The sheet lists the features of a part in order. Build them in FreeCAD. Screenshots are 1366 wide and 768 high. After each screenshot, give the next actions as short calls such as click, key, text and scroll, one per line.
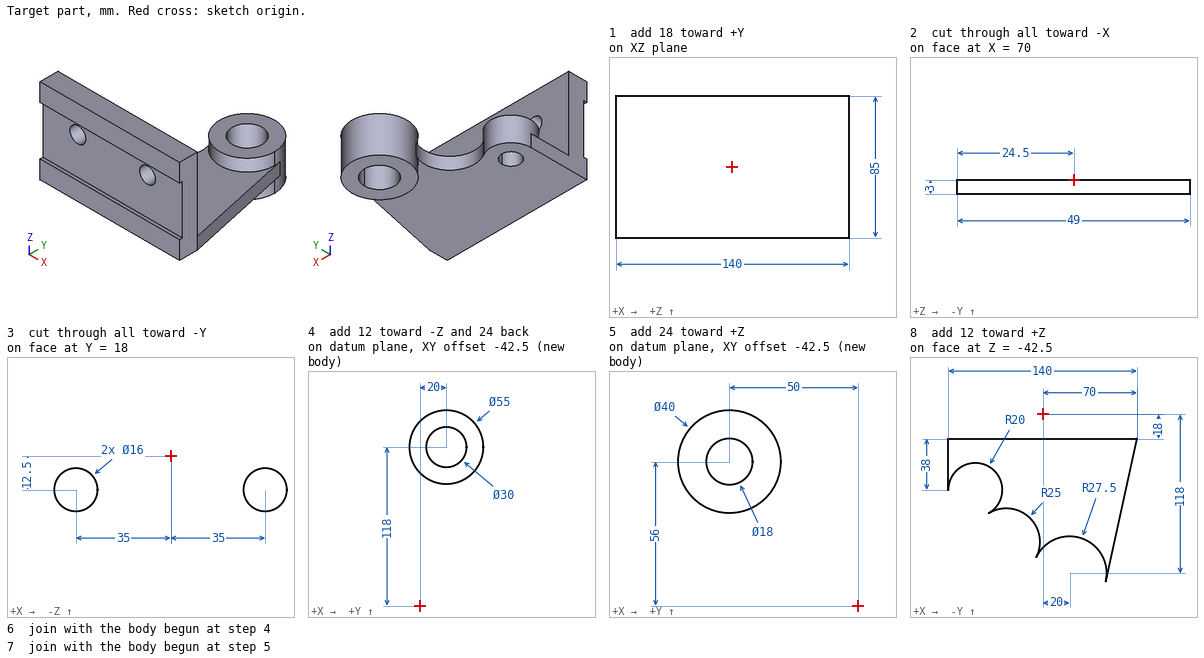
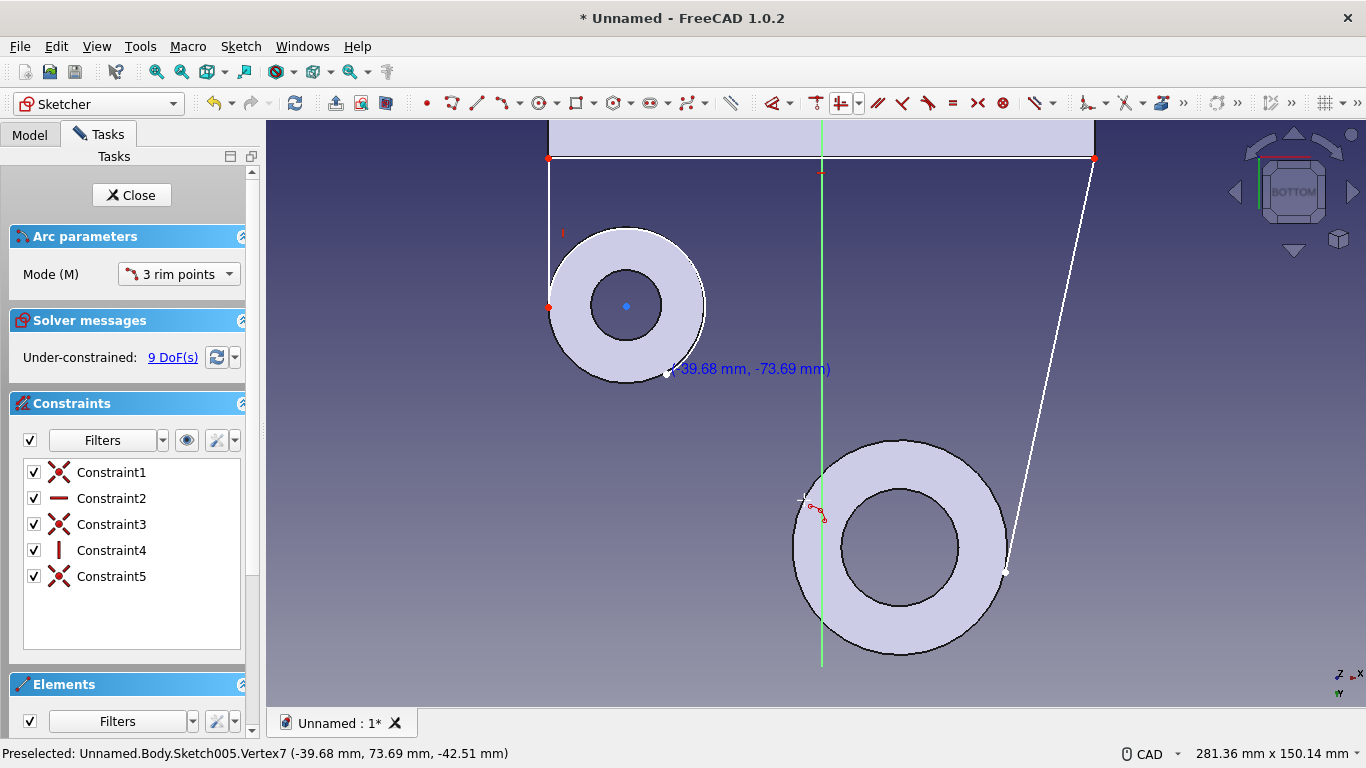
click(803, 500)
click(782, 385)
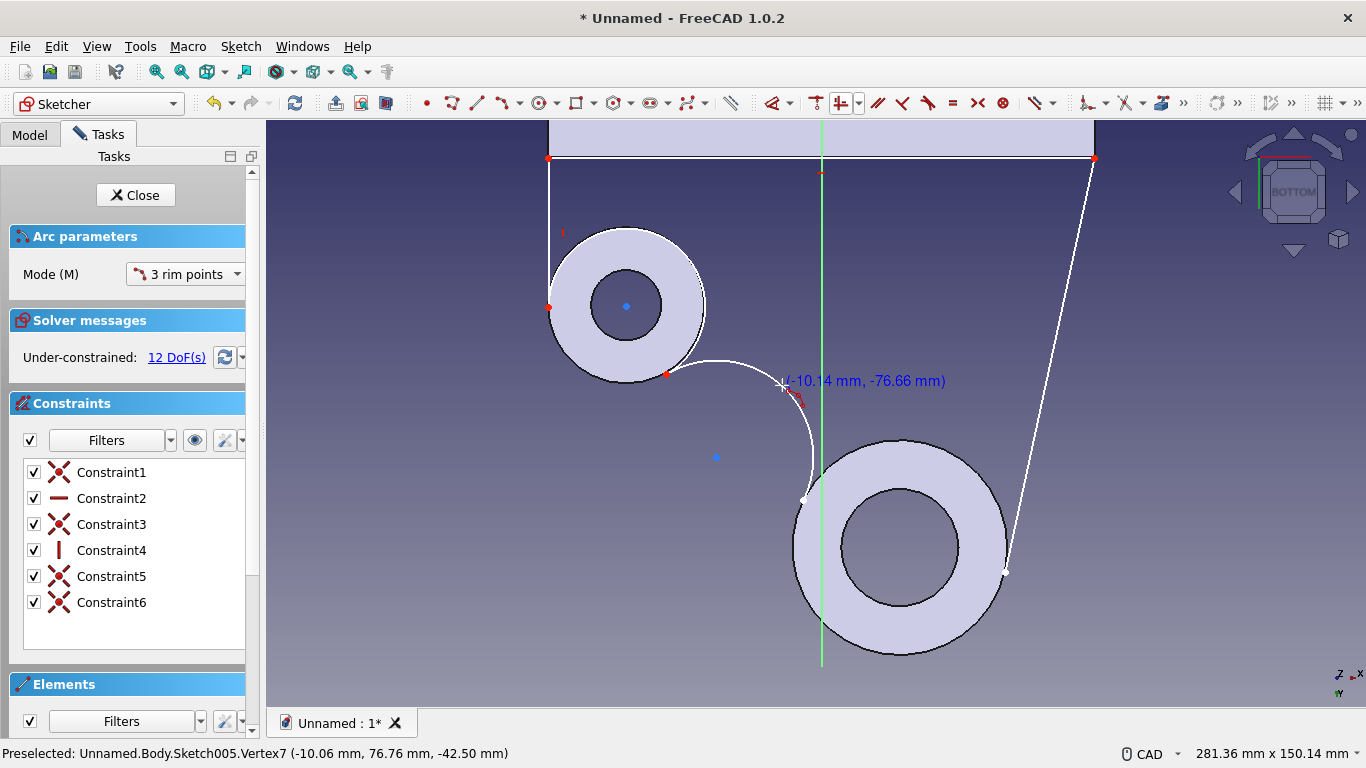
click(803, 501)
click(1005, 573)
click(935, 446)
key(Escape)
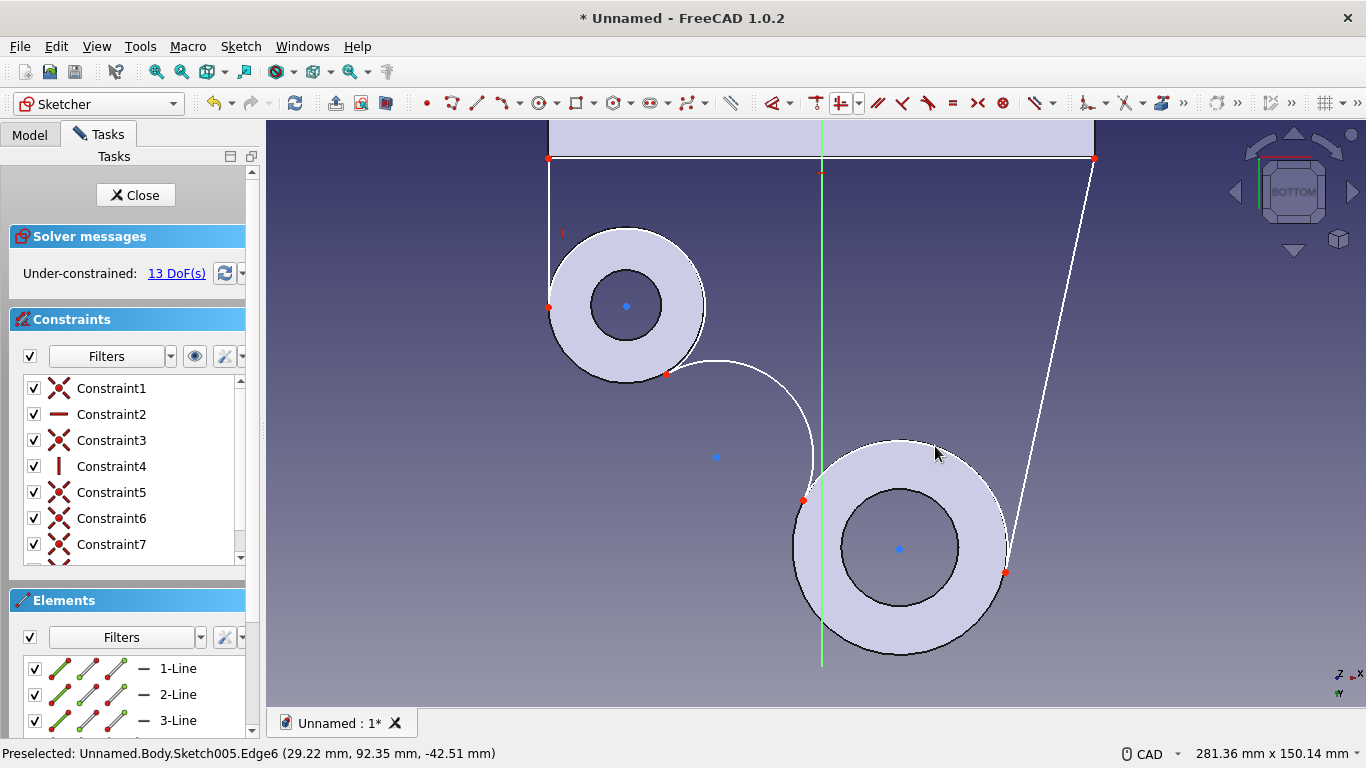
click(1032, 448)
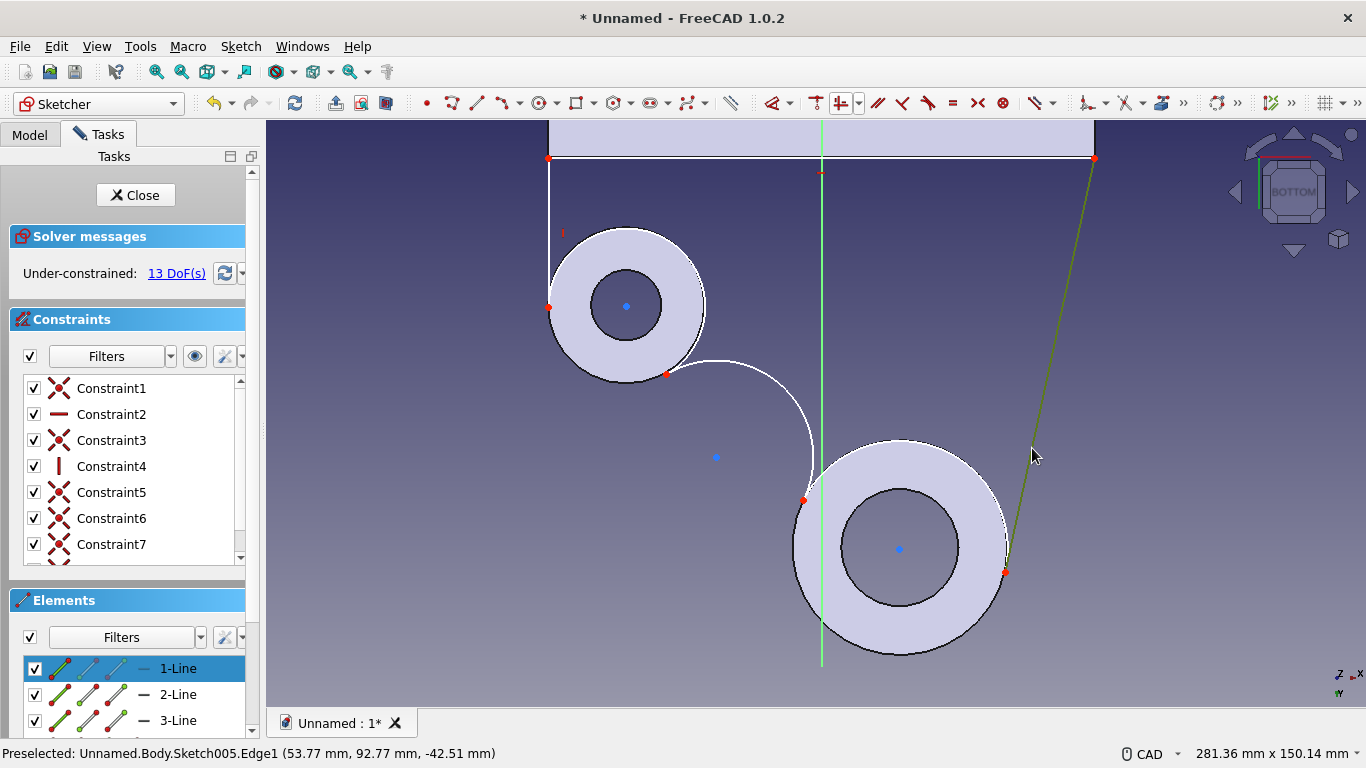
click(986, 484)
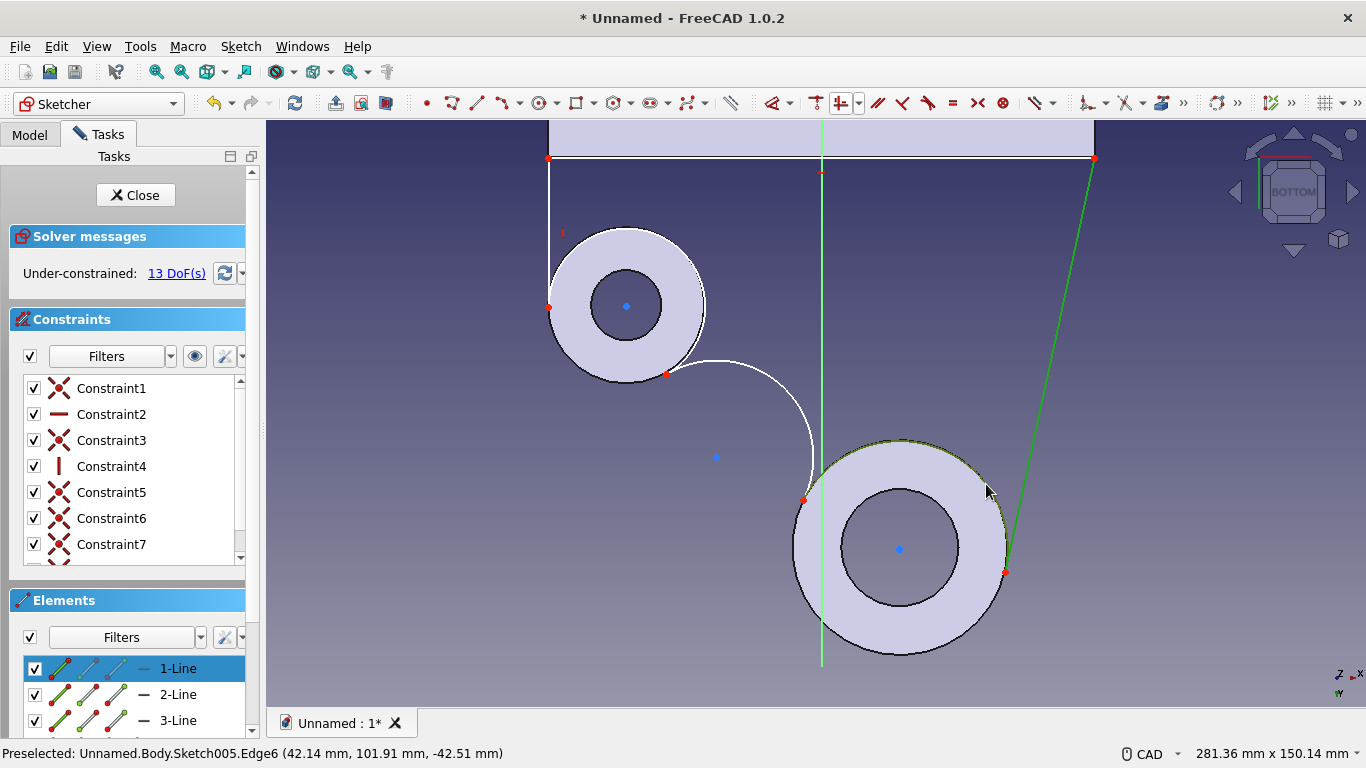
click(928, 104)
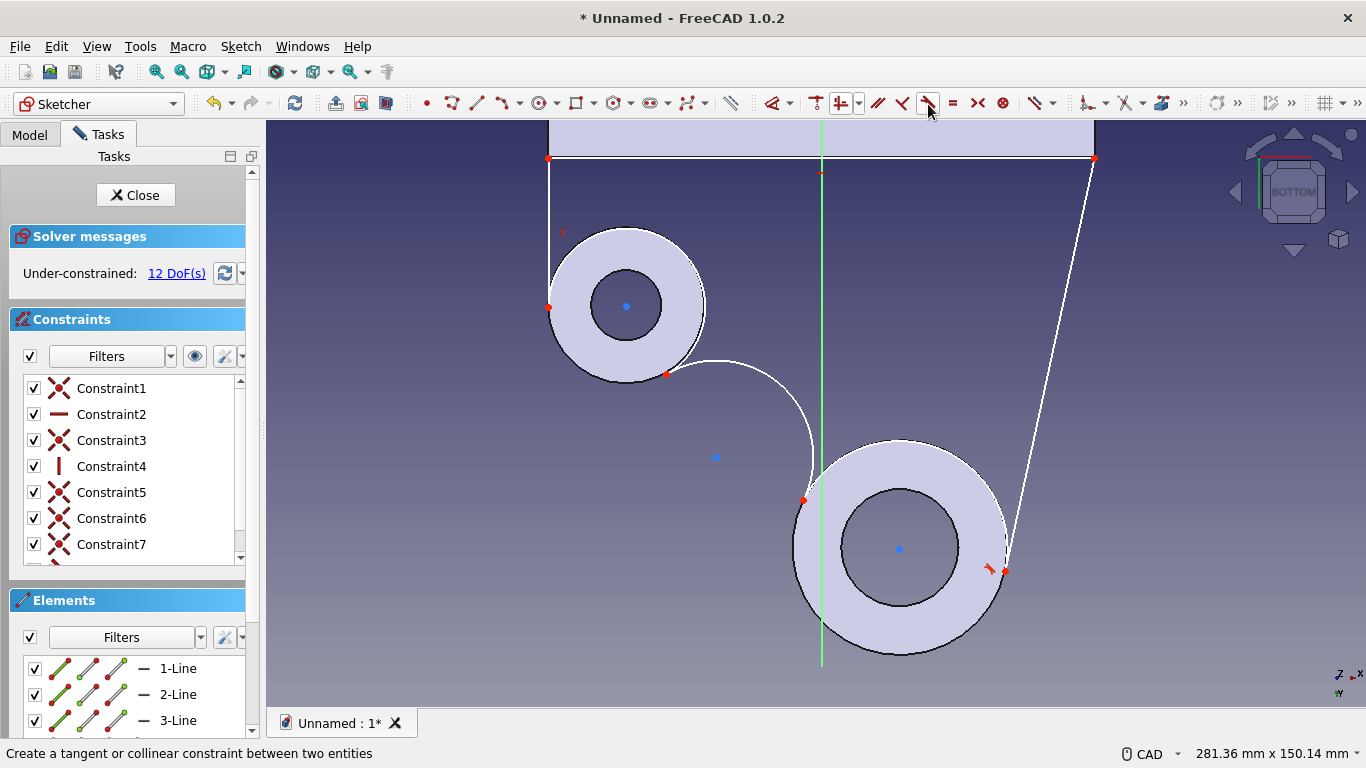
click(549, 203)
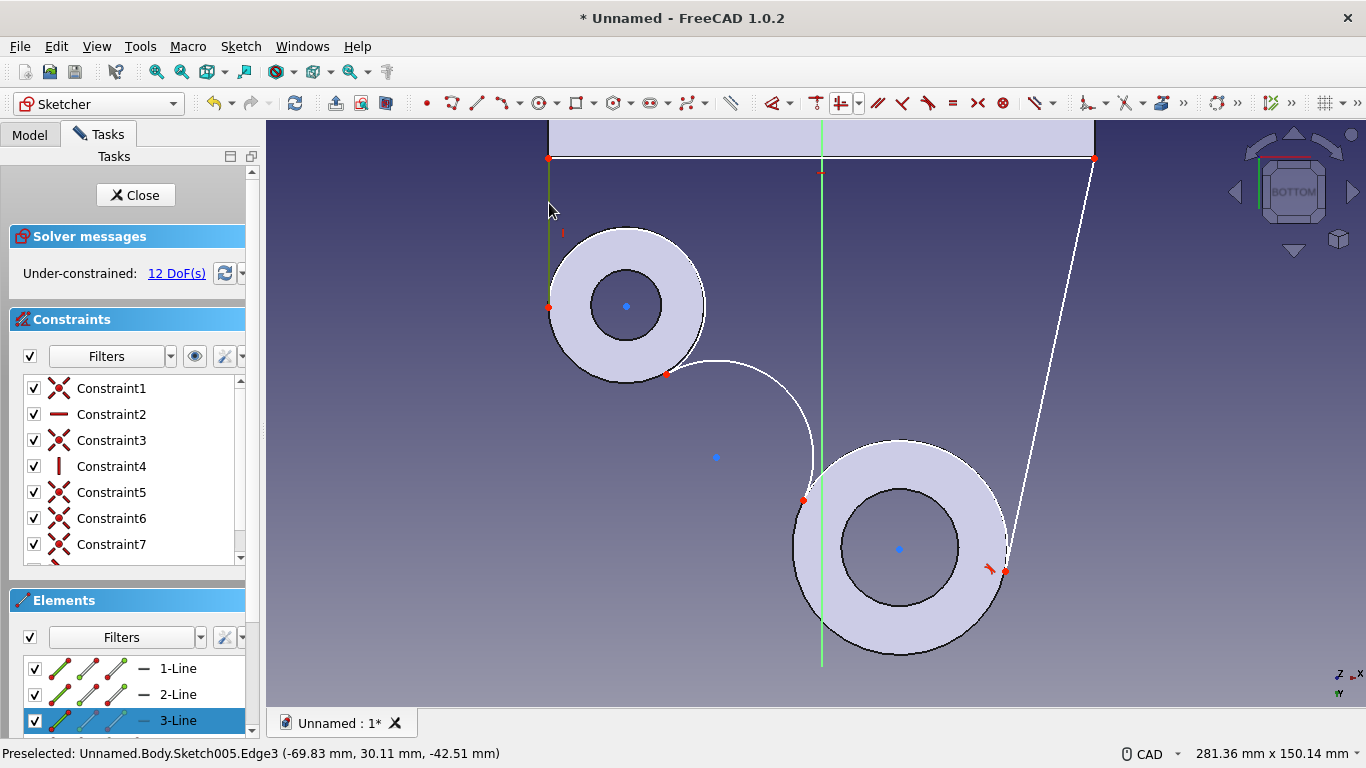
click(703, 290)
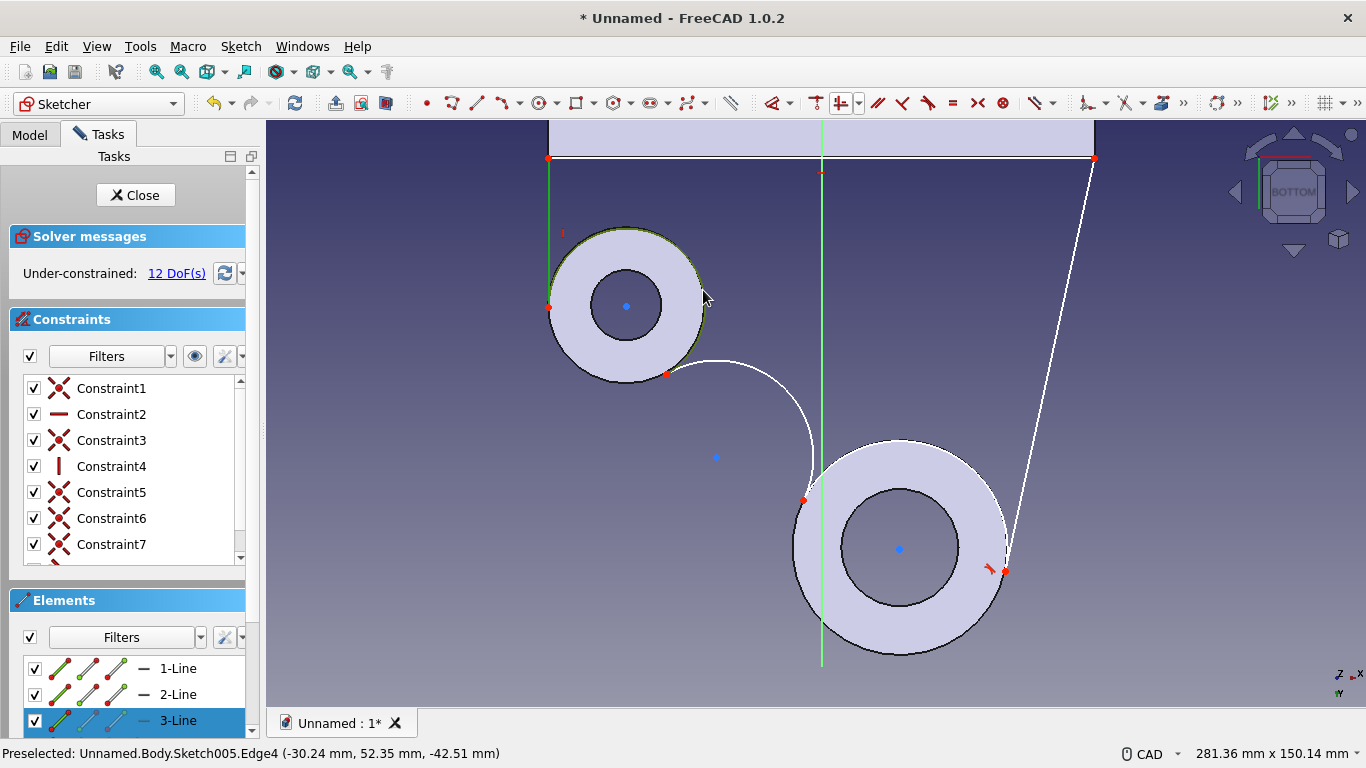
click(928, 104)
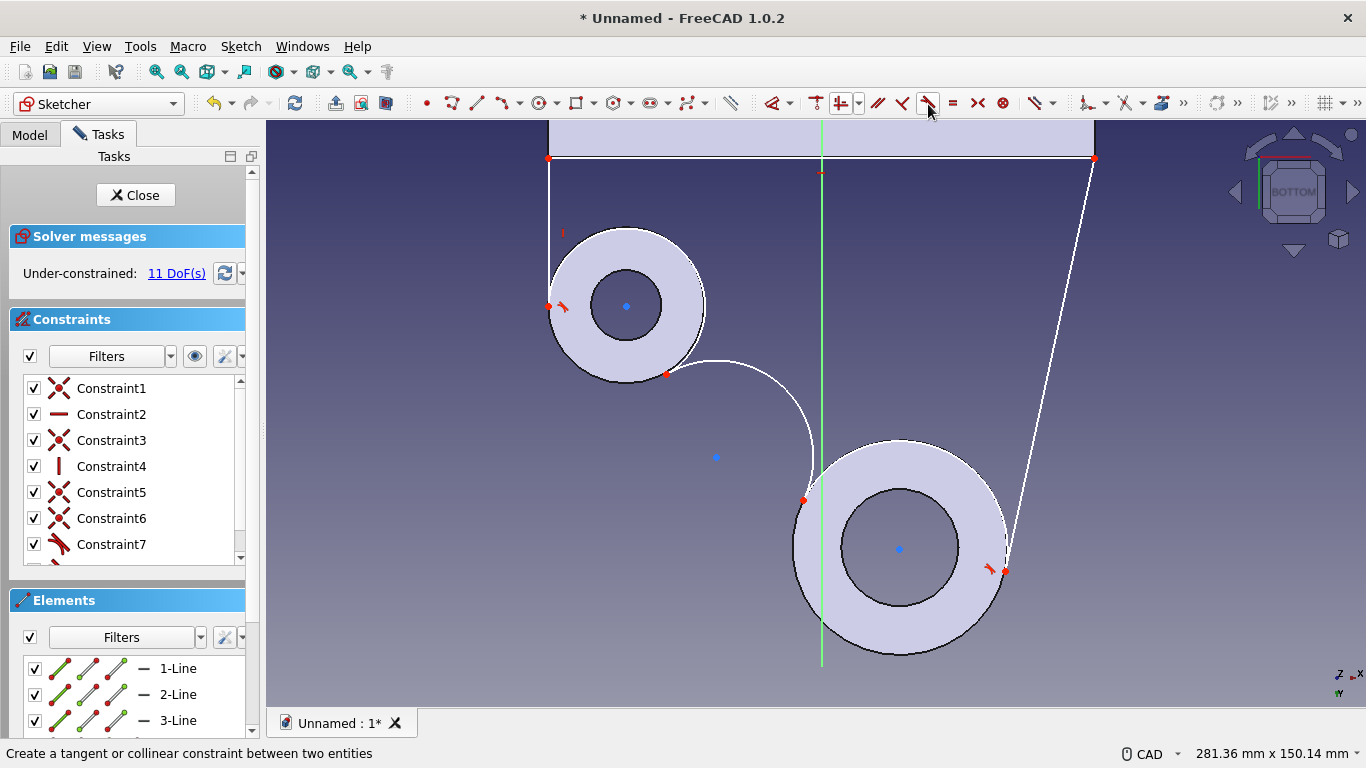
click(703, 290)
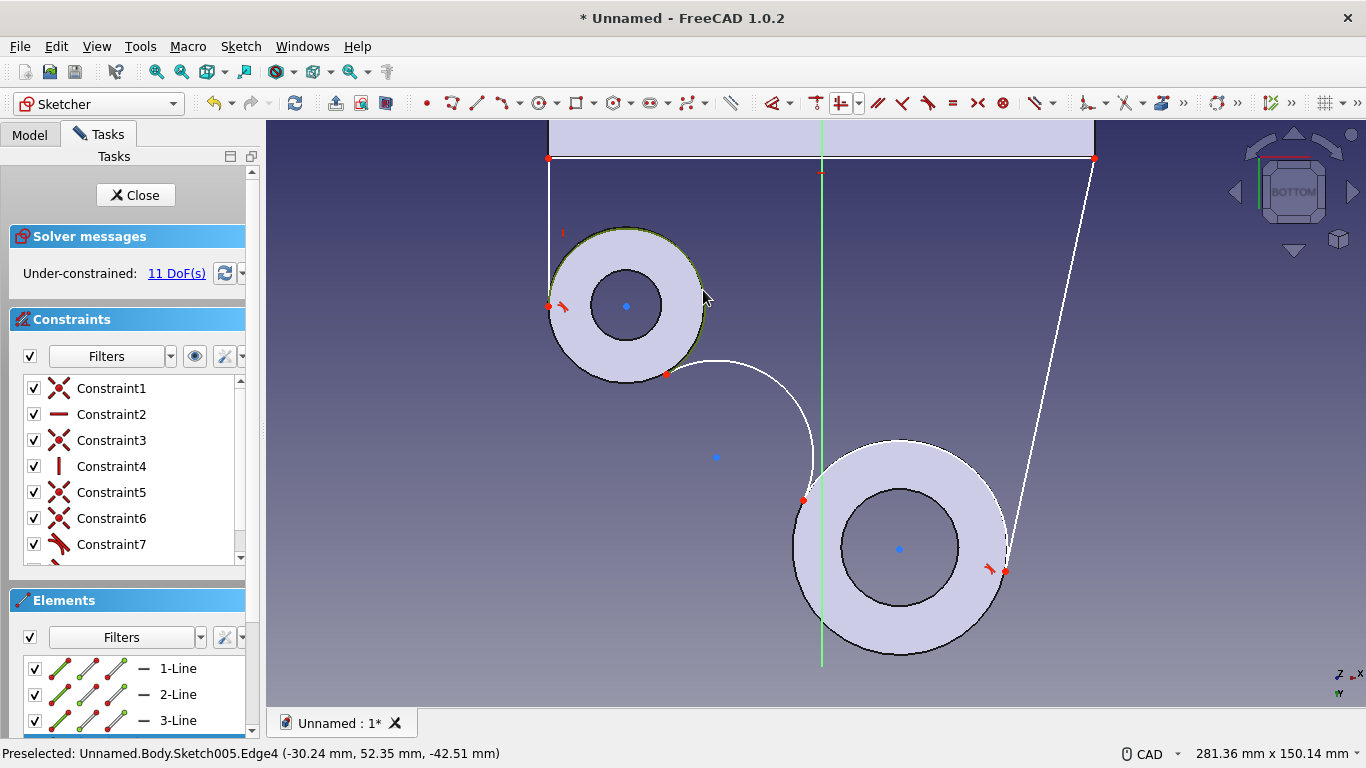
click(809, 428)